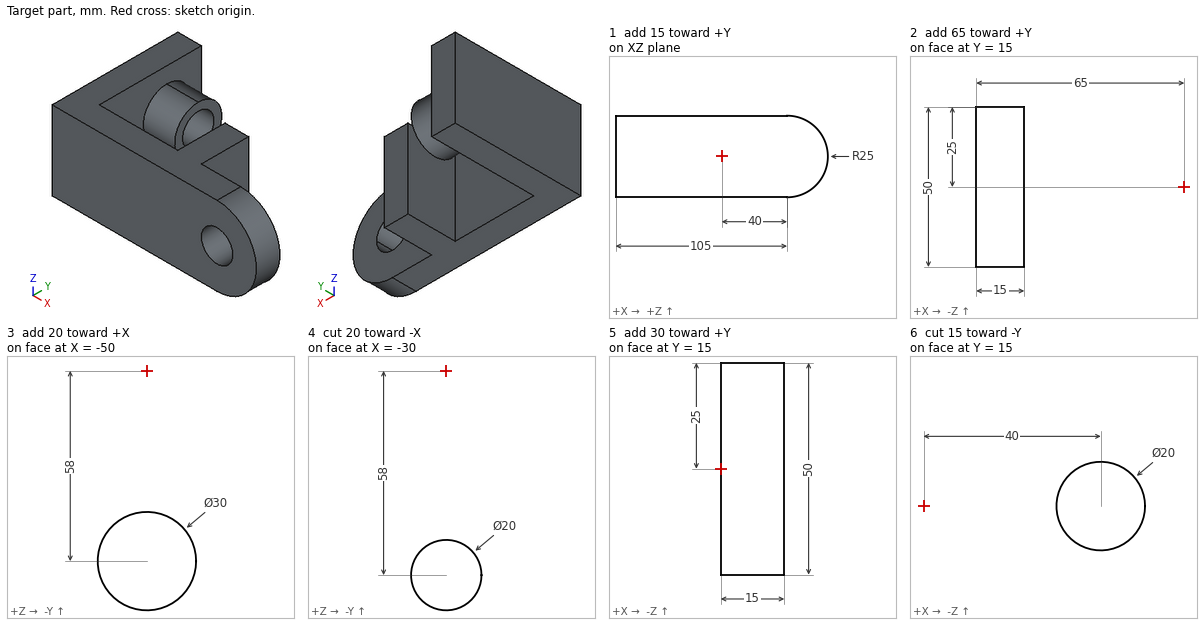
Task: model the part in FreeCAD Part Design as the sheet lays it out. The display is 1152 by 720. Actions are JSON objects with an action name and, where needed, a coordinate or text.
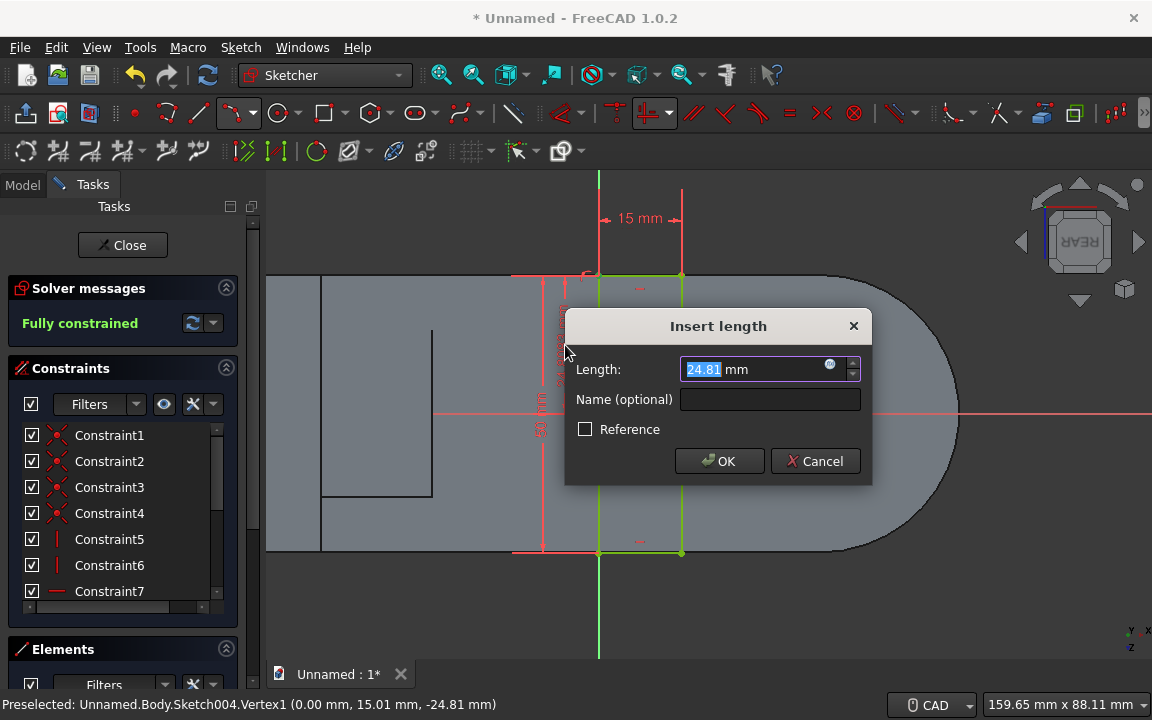
{"action": "type", "text": "25"}
{"action": "key", "text": "Return"}
{"action": "key", "text": "Escape"}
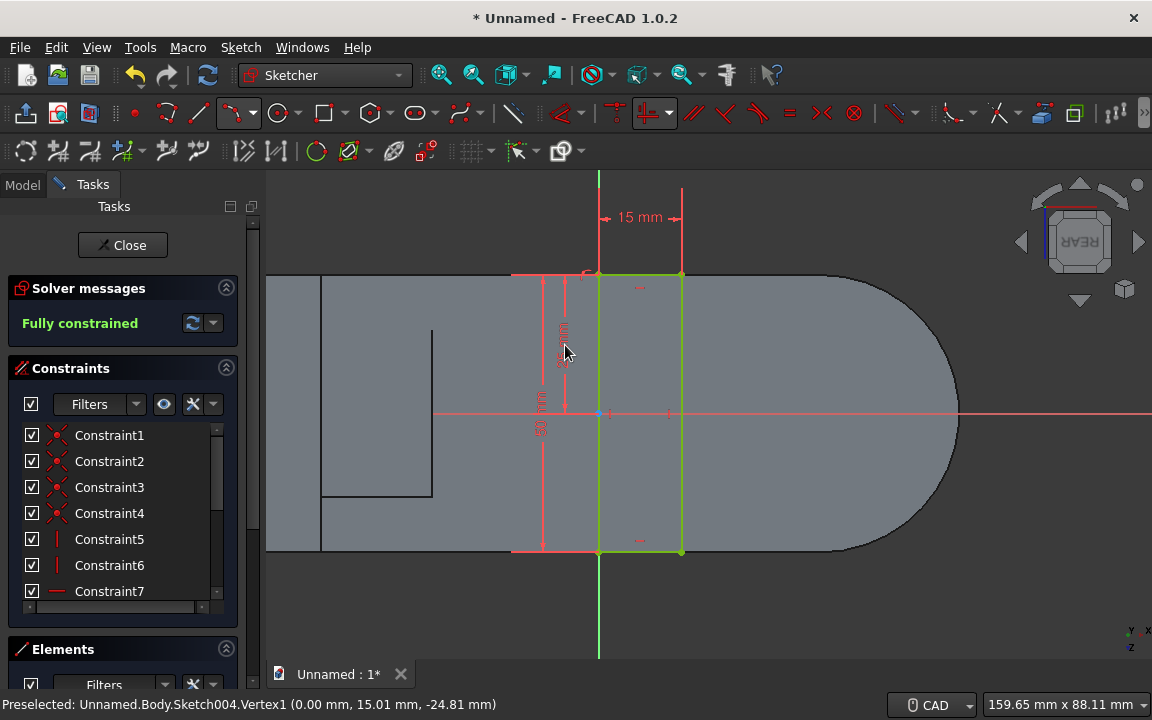
{"action": "left_click", "coordinate": [123, 245]}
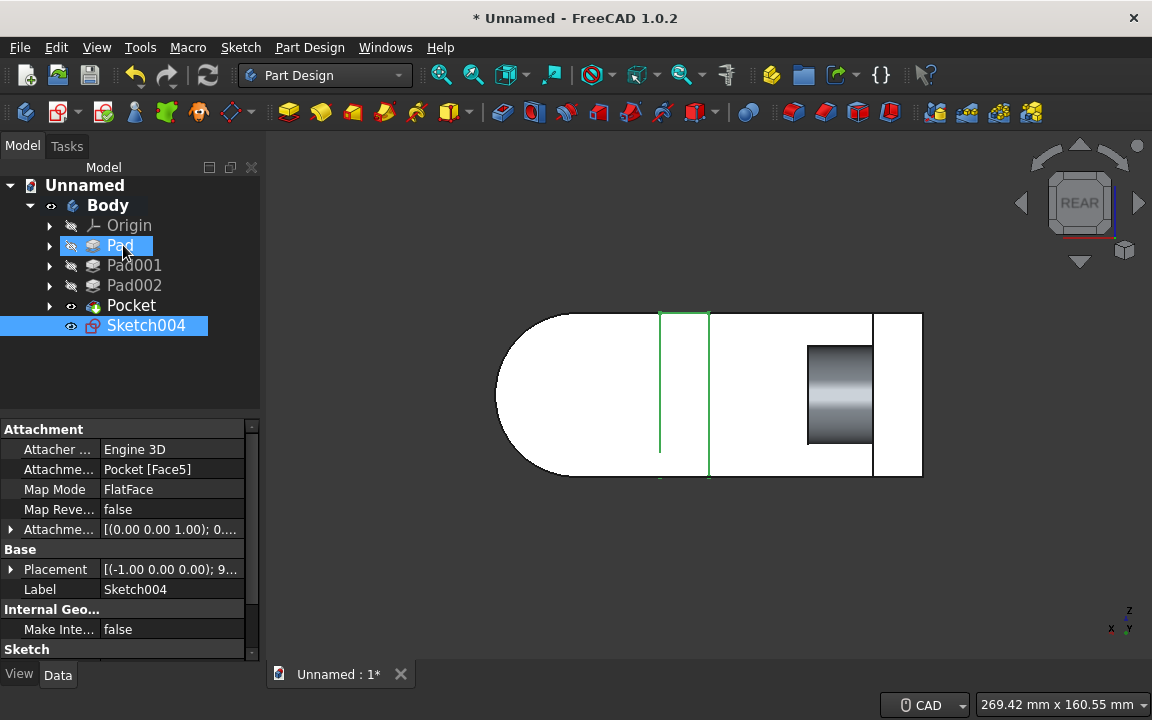
{"action": "left_click", "coordinate": [290, 112]}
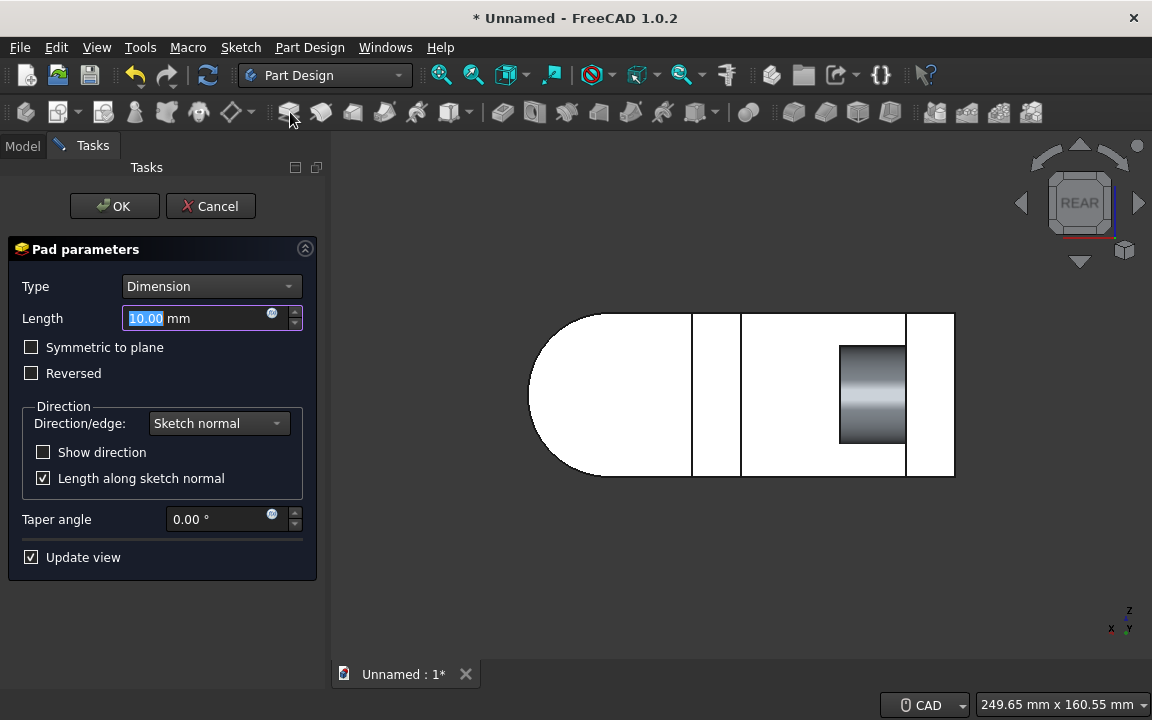
{"action": "type", "text": "30"}
{"action": "key", "text": "Tab"}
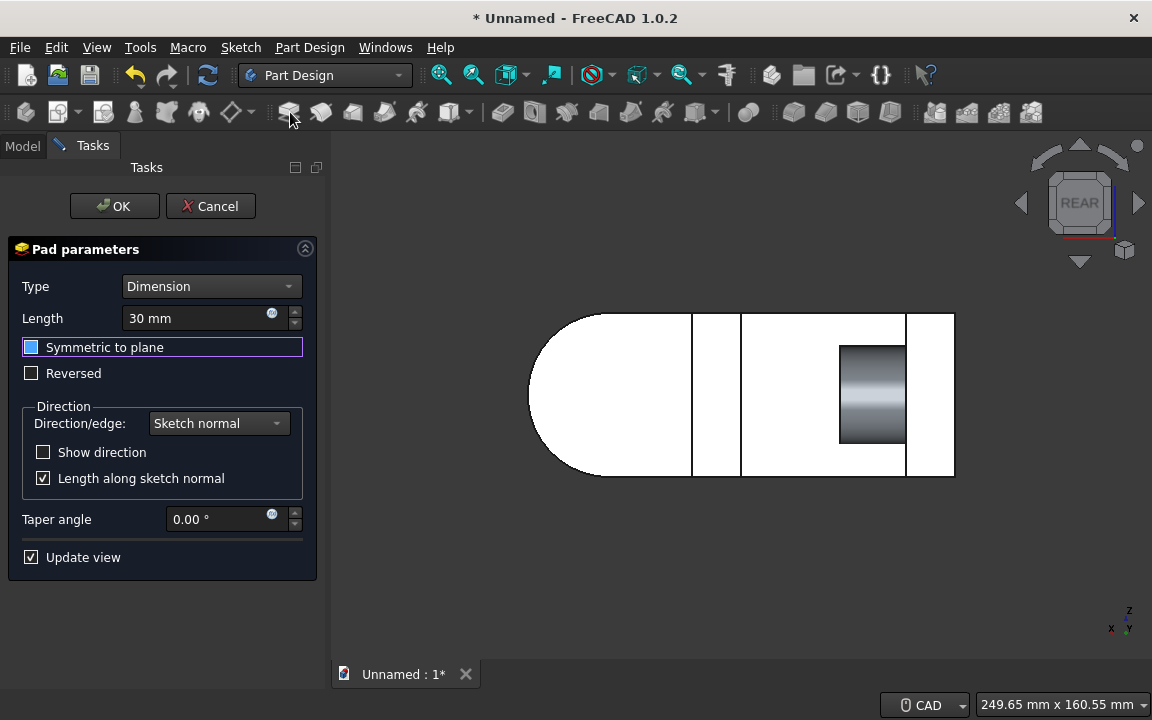
{"action": "left_click", "coordinate": [115, 206]}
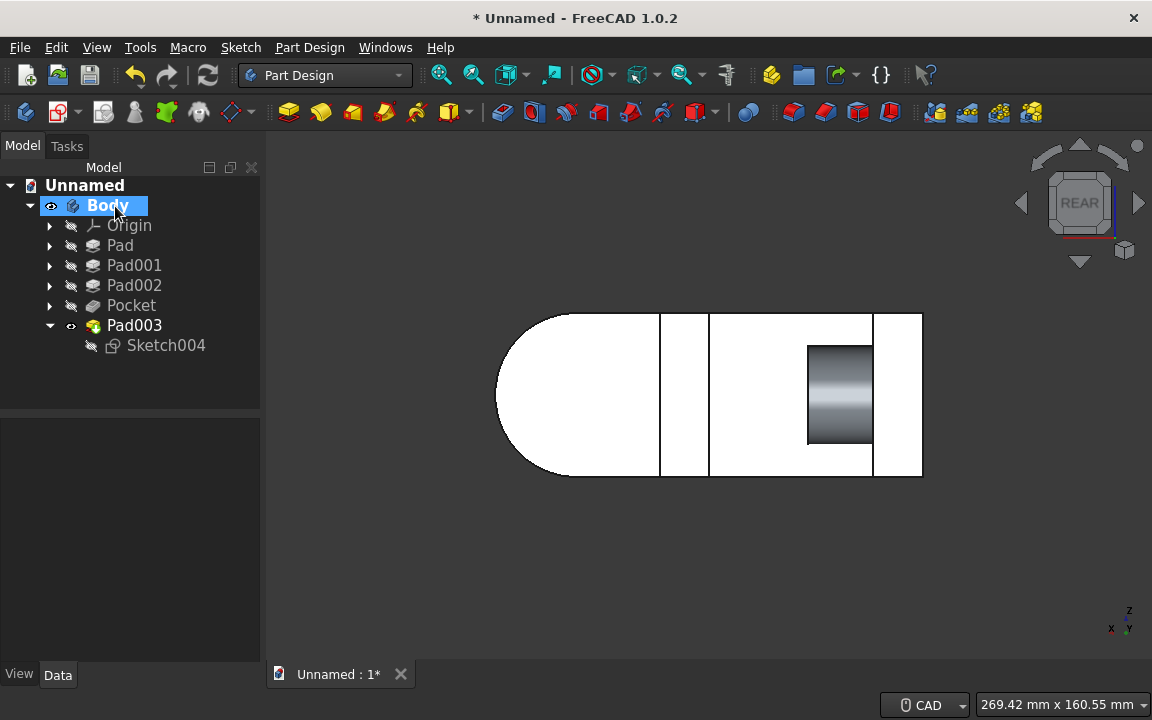
{"action": "left_click", "coordinate": [791, 394]}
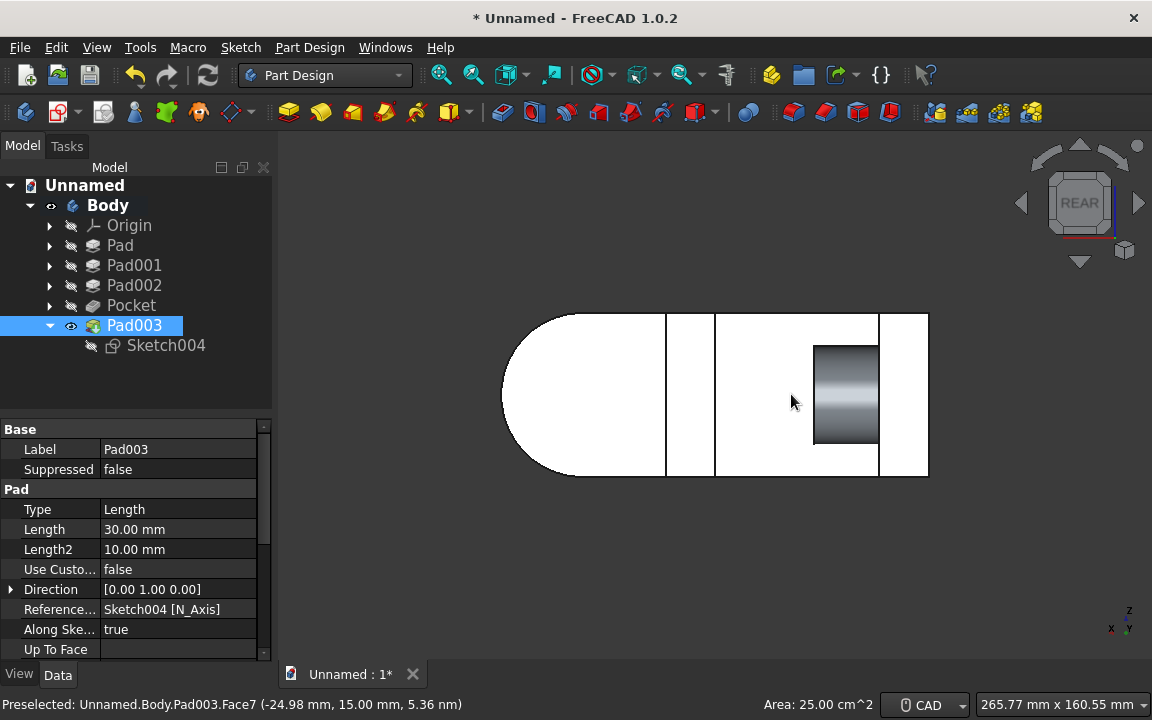
{"action": "left_click", "coordinate": [58, 112]}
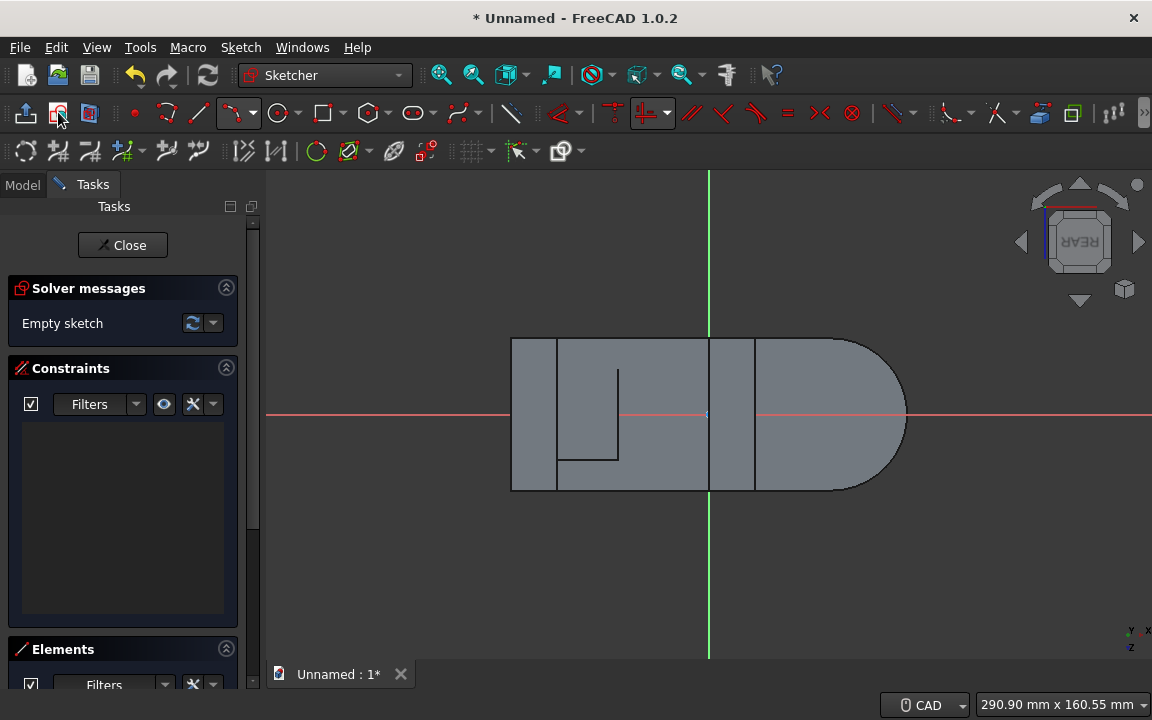
{"action": "scroll", "coordinate": [879, 414], "scroll_direction": "up", "scroll_amount": 8}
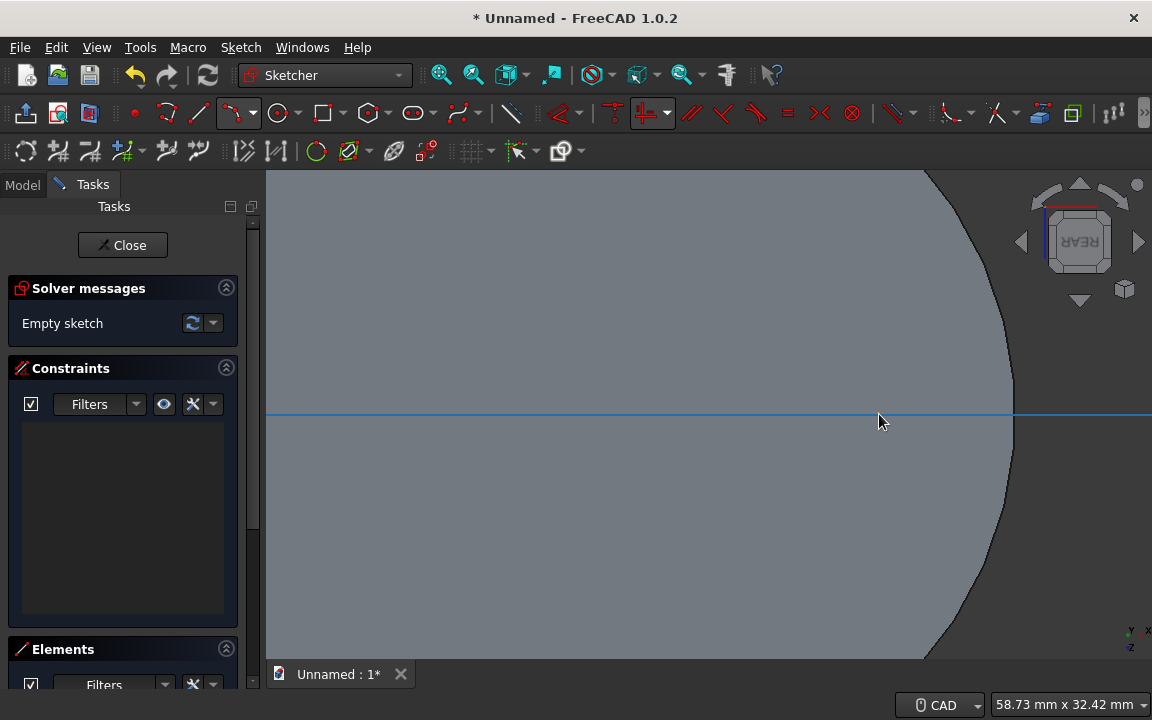
{"action": "left_click", "coordinate": [278, 114]}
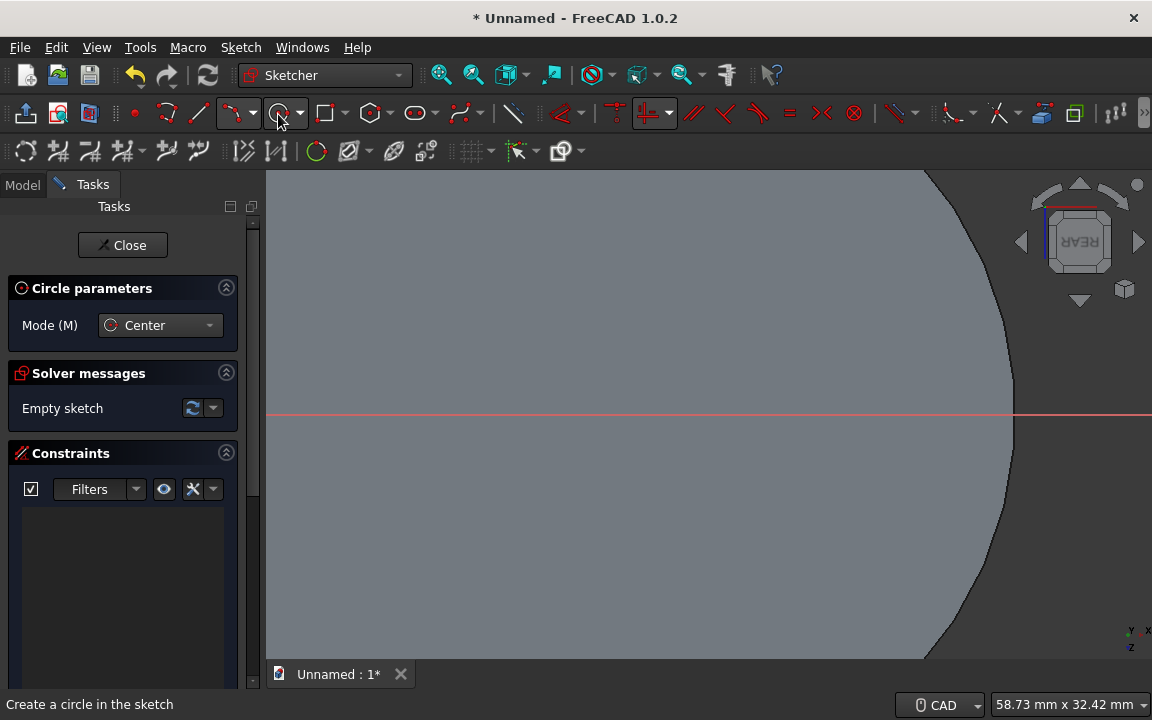
{"action": "left_click", "coordinate": [638, 414]}
{"action": "mouse_move", "coordinate": [745, 308]}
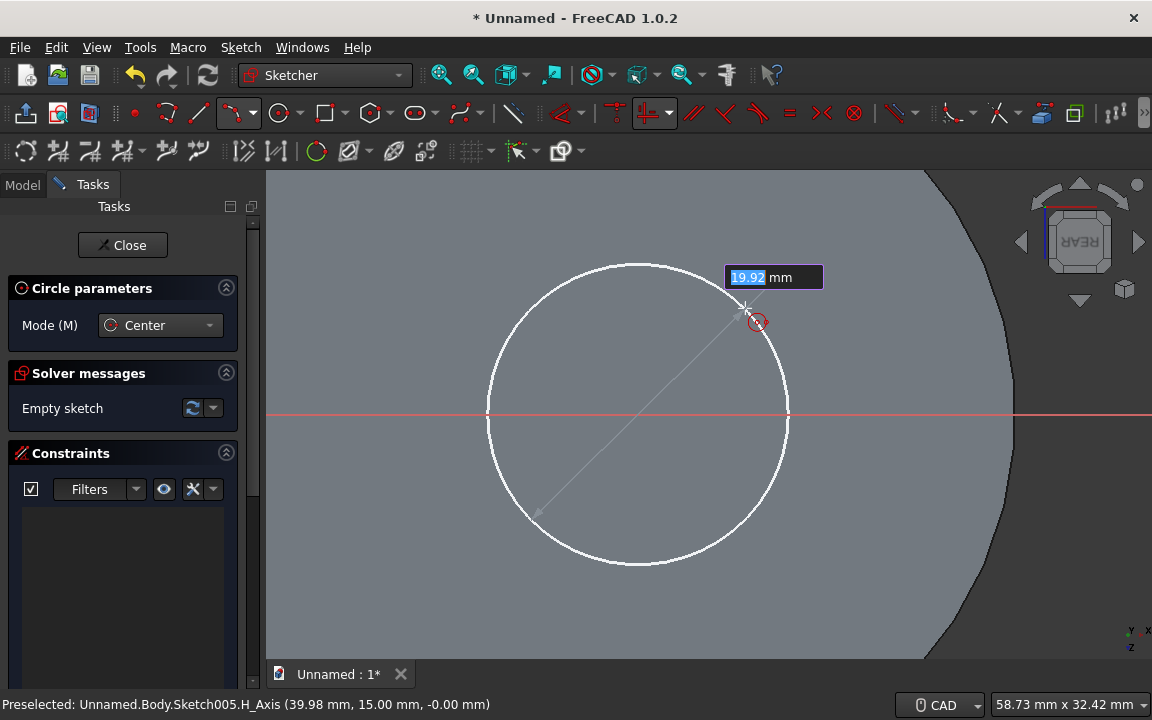
{"action": "type", "text": "20"}
{"action": "key", "text": "Return"}
{"action": "key", "text": "Escape"}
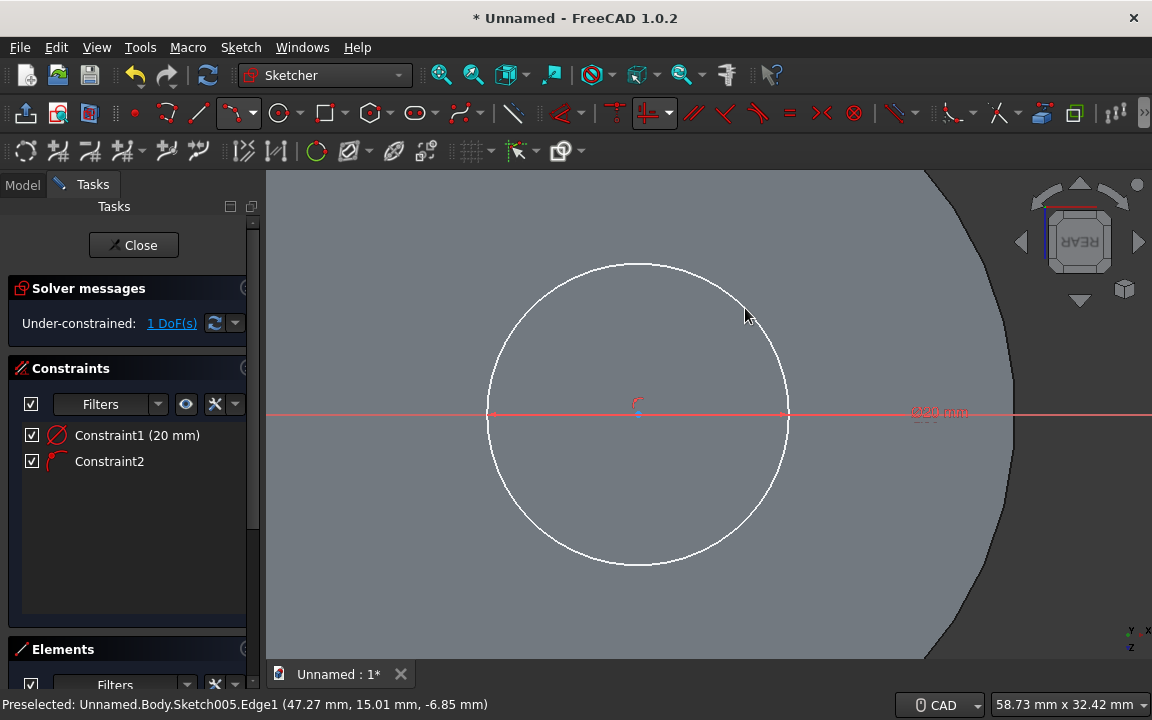
{"action": "left_click", "coordinate": [560, 114]}